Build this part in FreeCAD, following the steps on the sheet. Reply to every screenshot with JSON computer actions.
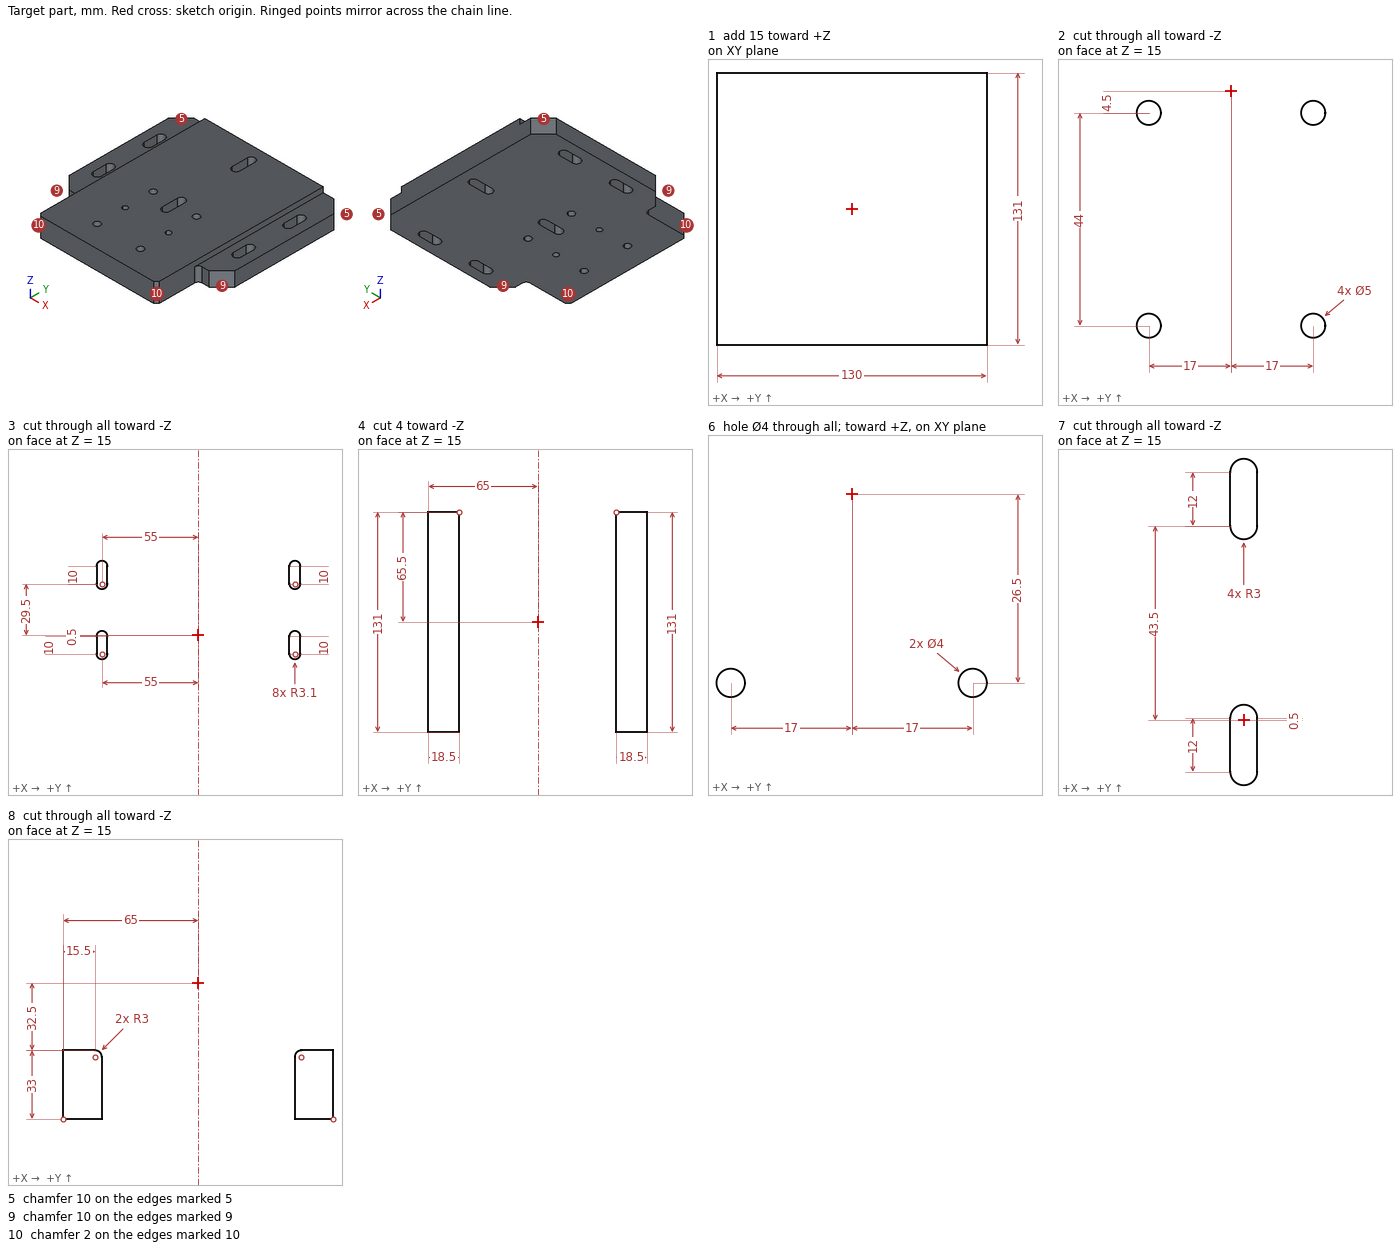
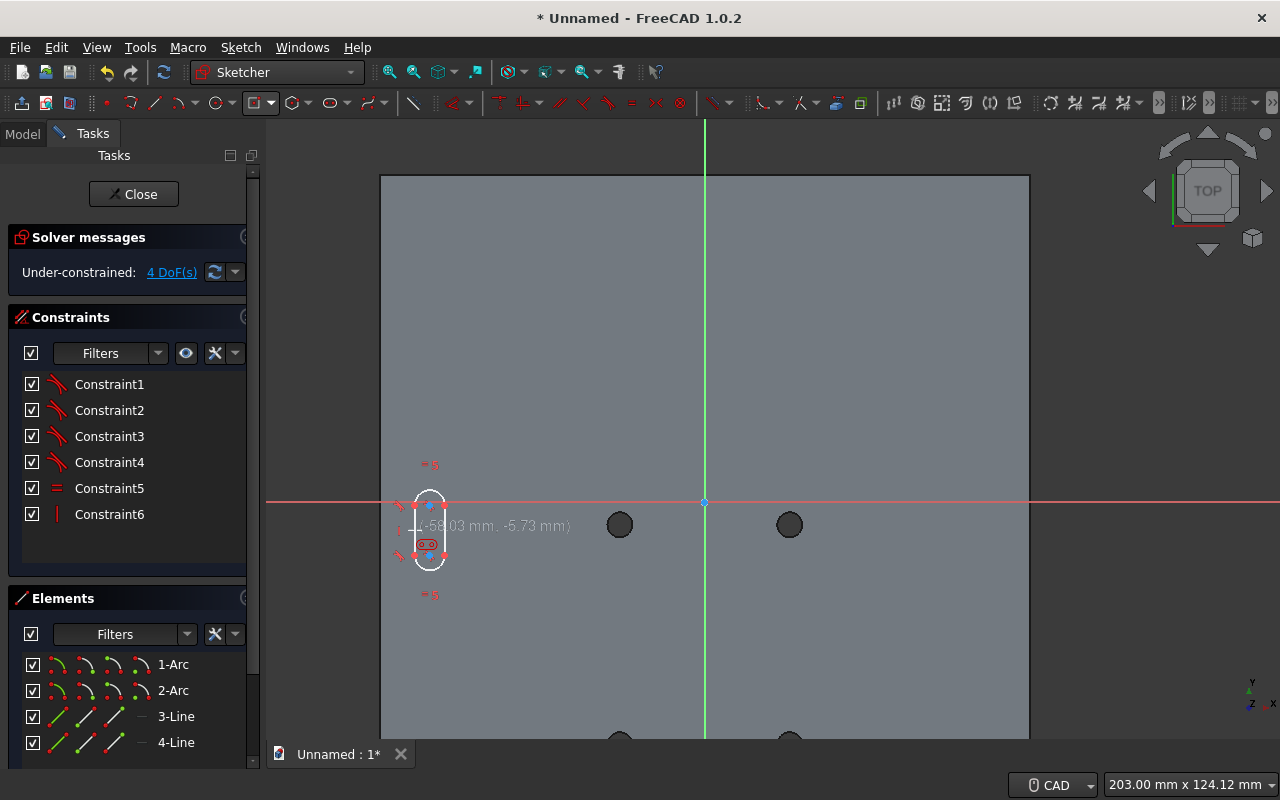
{"action": "scroll", "coordinate": [430, 355], "scroll_direction": "up", "scroll_amount": 2}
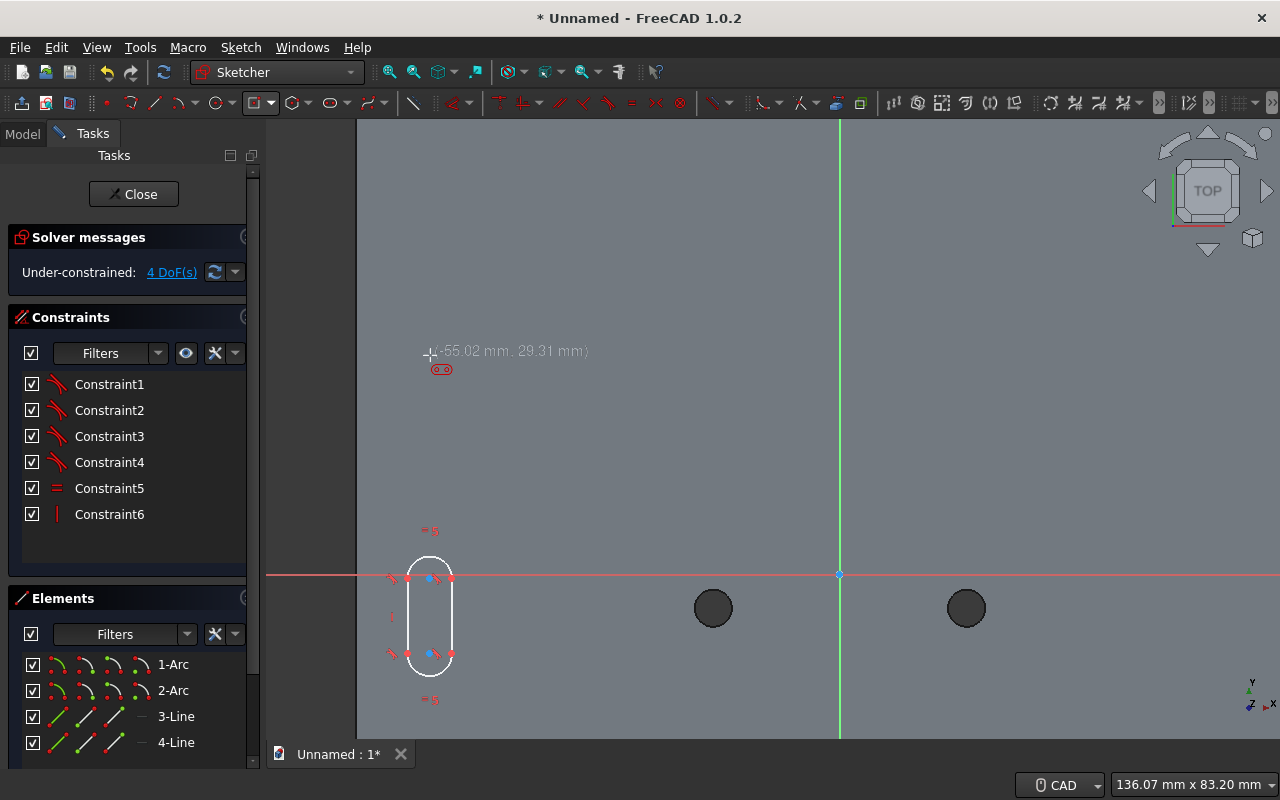
{"action": "left_click", "coordinate": [430, 355]}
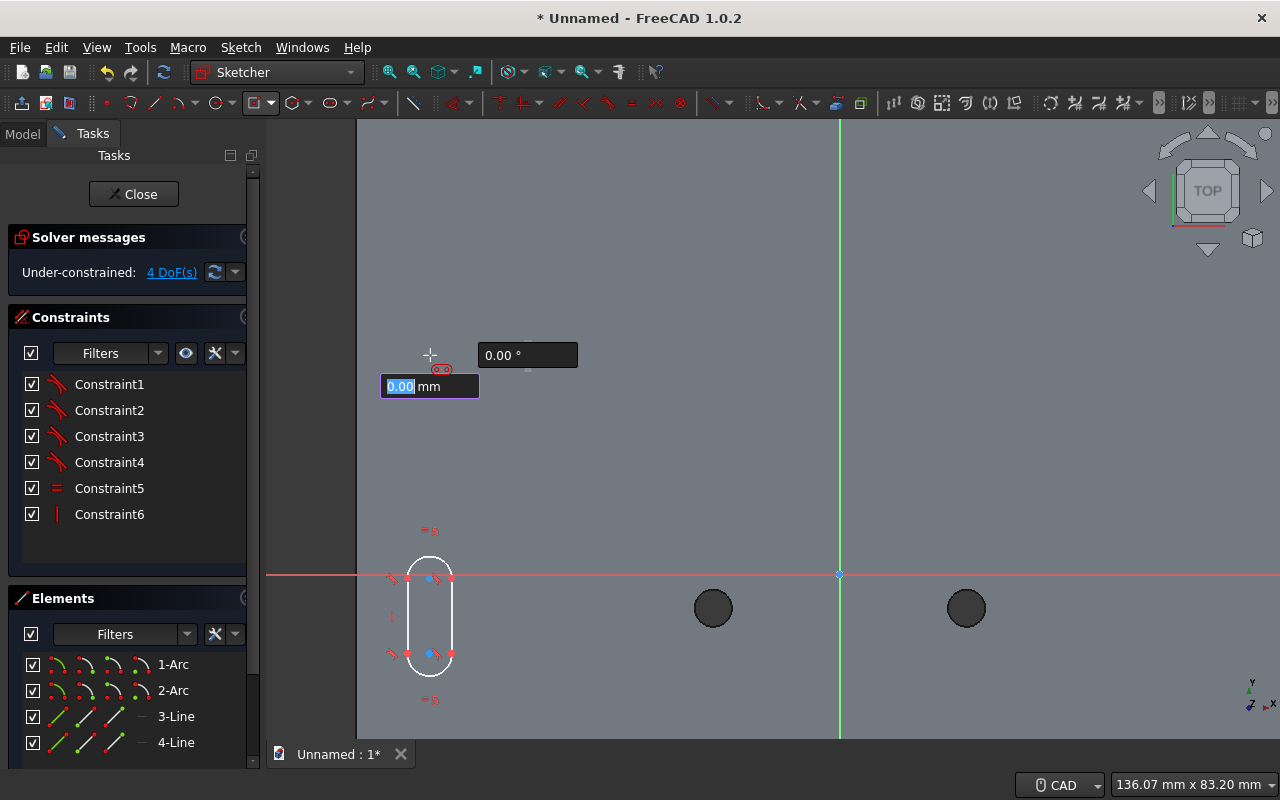
{"action": "left_click", "coordinate": [430, 280]}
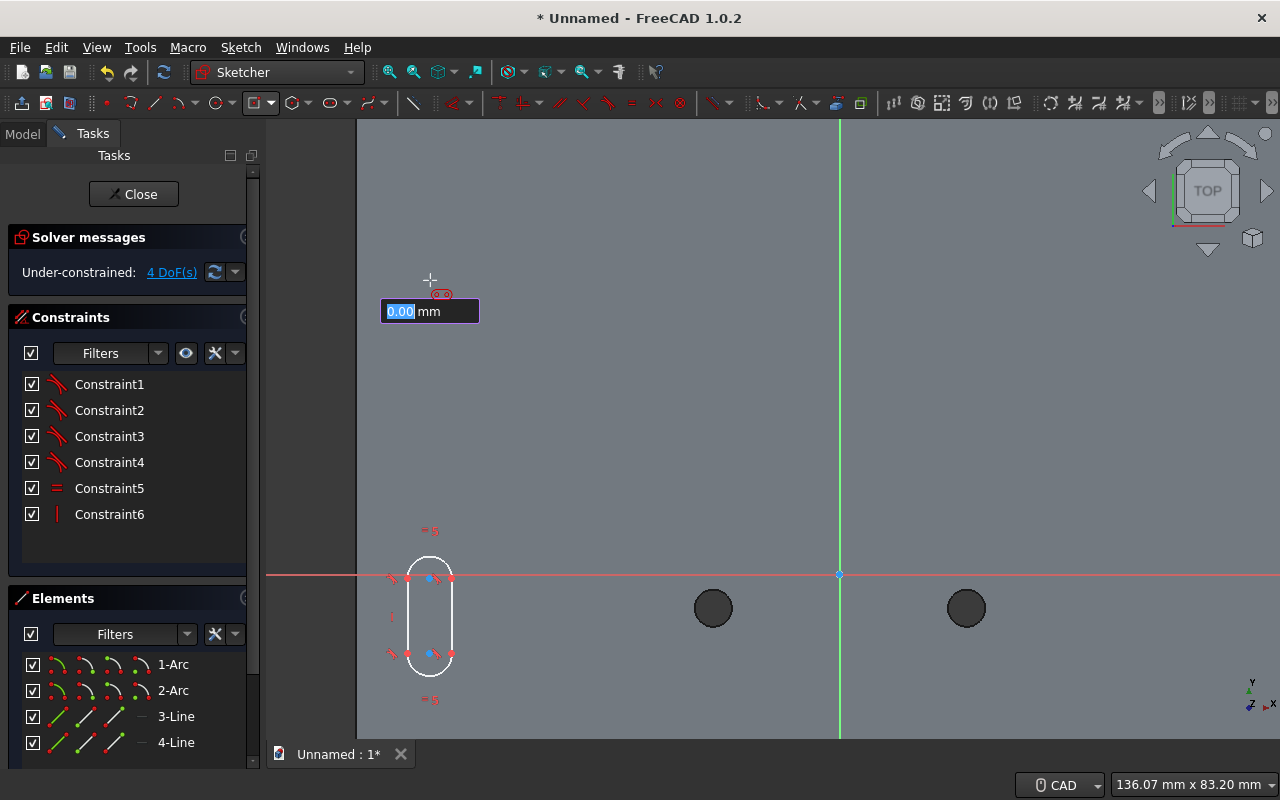
{"action": "left_click", "coordinate": [407, 318]}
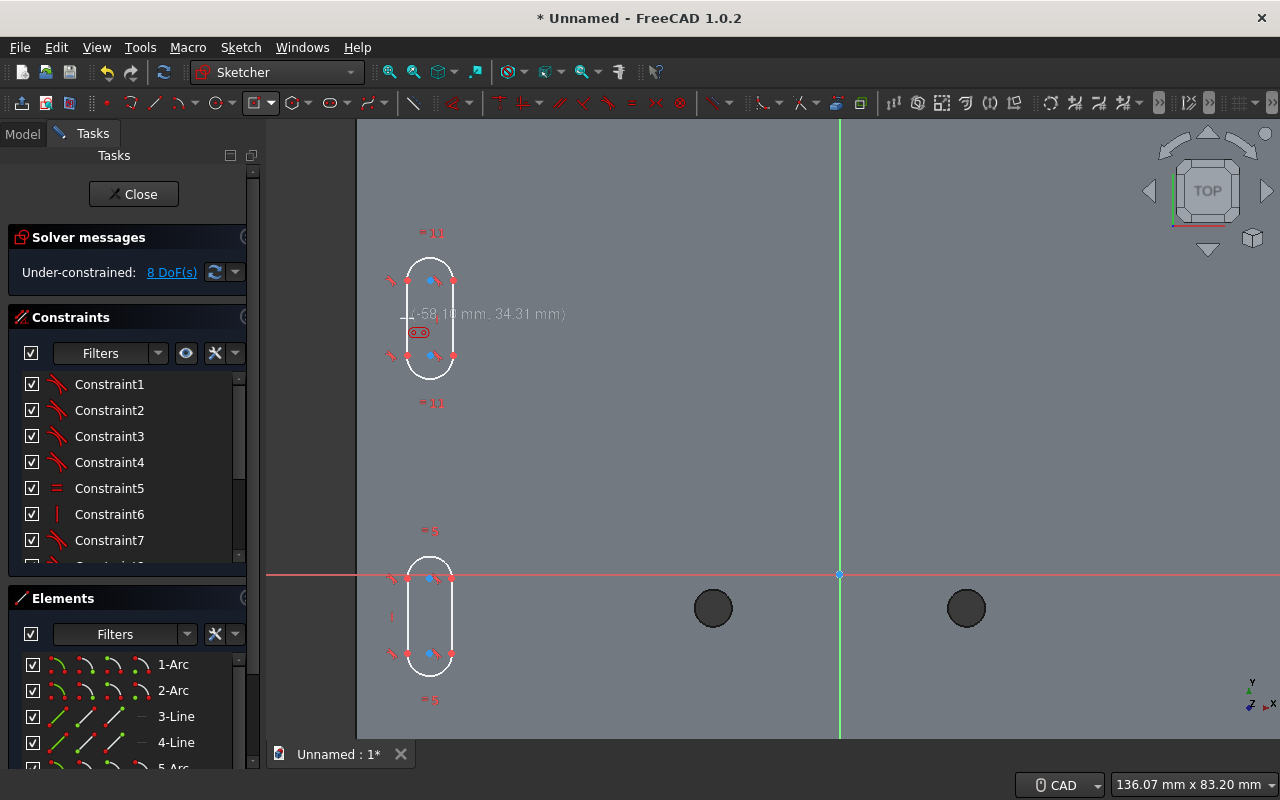
{"action": "scroll", "coordinate": [429, 352], "scroll_direction": "down", "scroll_amount": 2}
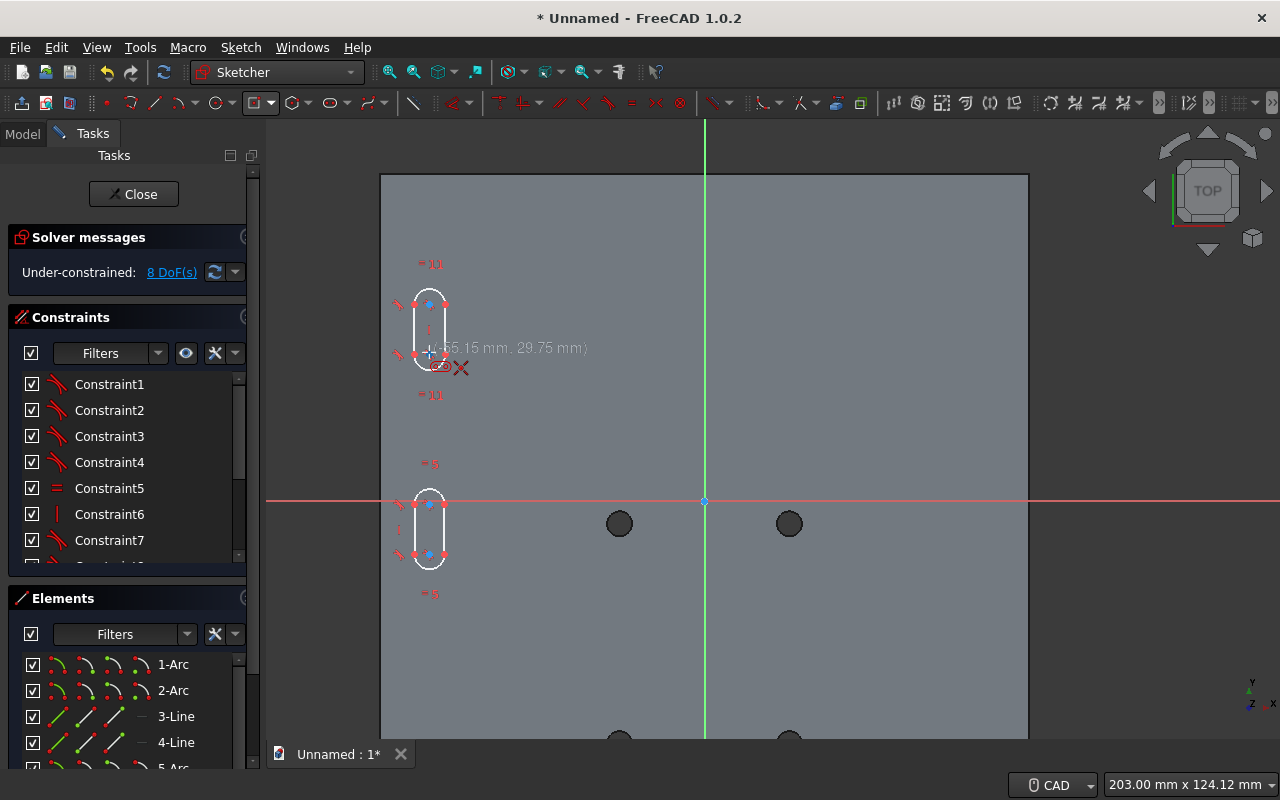
{"action": "scroll", "coordinate": [979, 554], "scroll_direction": "up", "scroll_amount": 2}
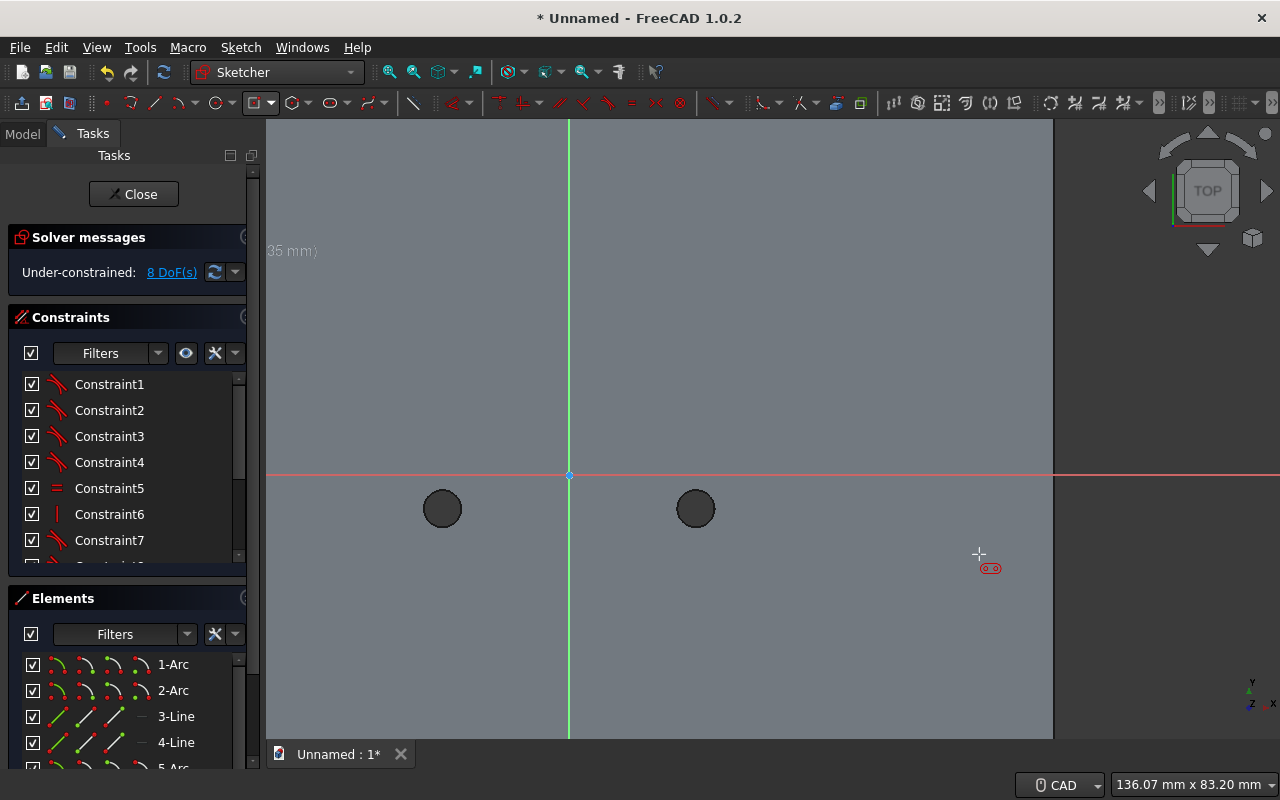
{"action": "left_click", "coordinate": [979, 553]}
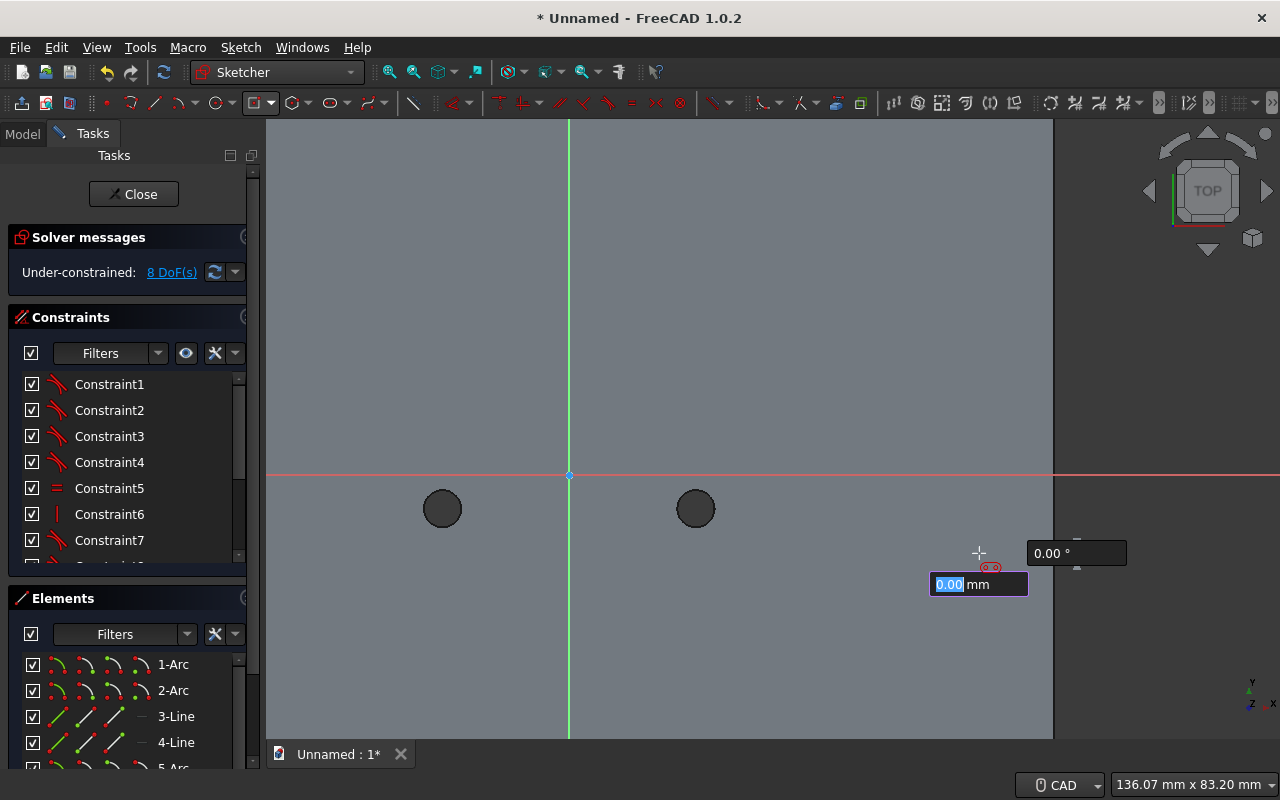
{"action": "scroll", "coordinate": [979, 479], "scroll_direction": "up", "scroll_amount": 8}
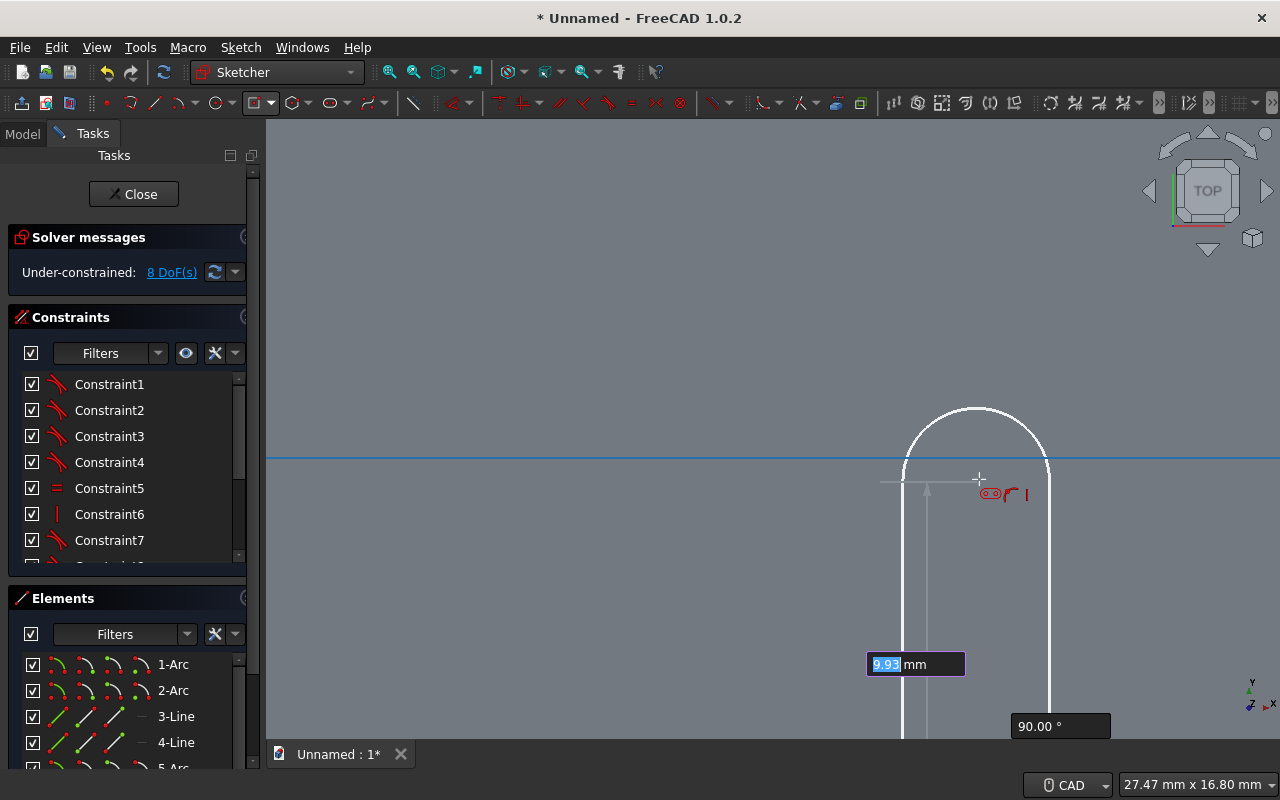
{"action": "left_click", "coordinate": [976, 476]}